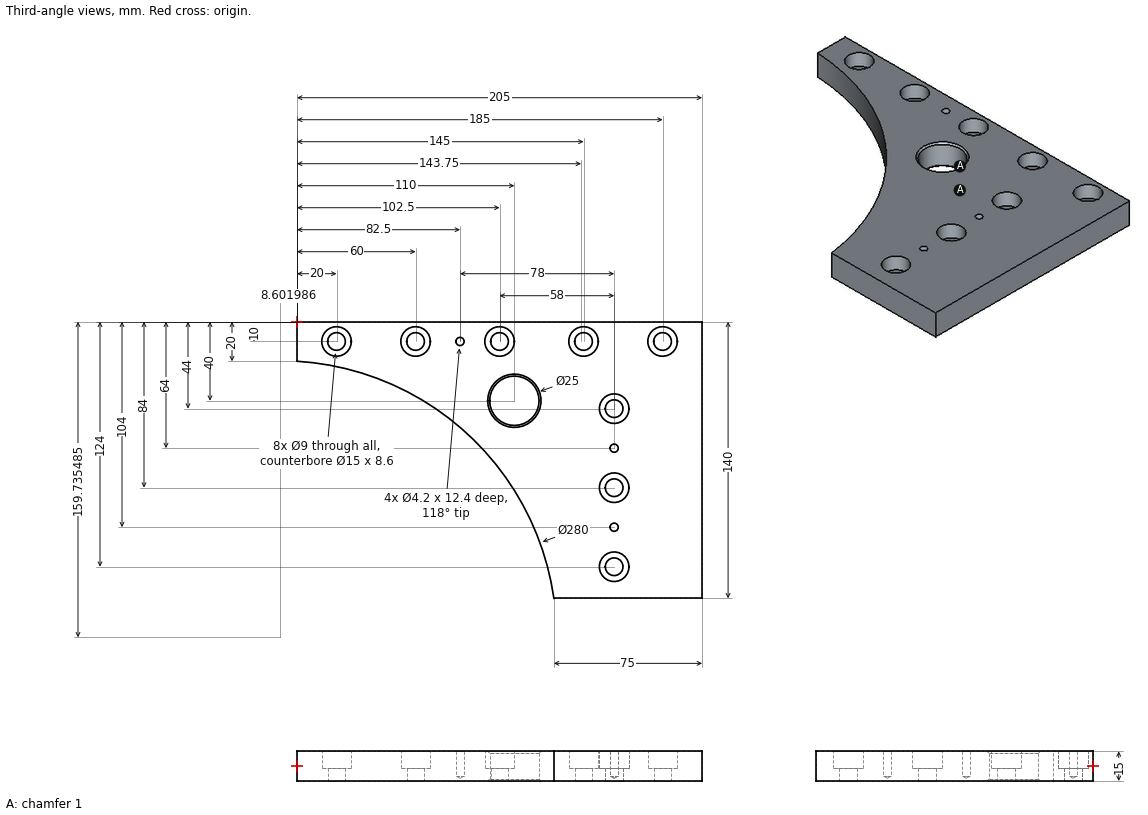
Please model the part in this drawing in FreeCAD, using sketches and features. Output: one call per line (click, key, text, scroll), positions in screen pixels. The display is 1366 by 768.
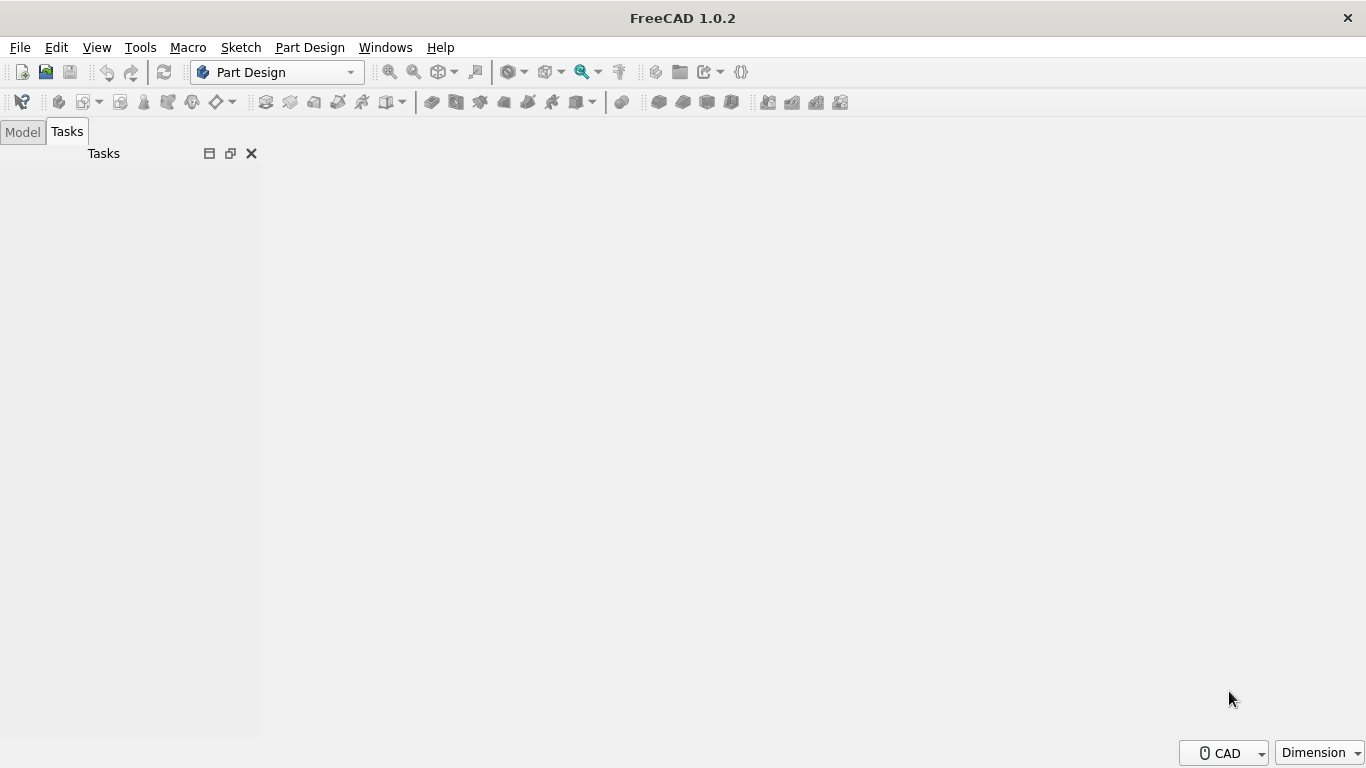
click(22, 72)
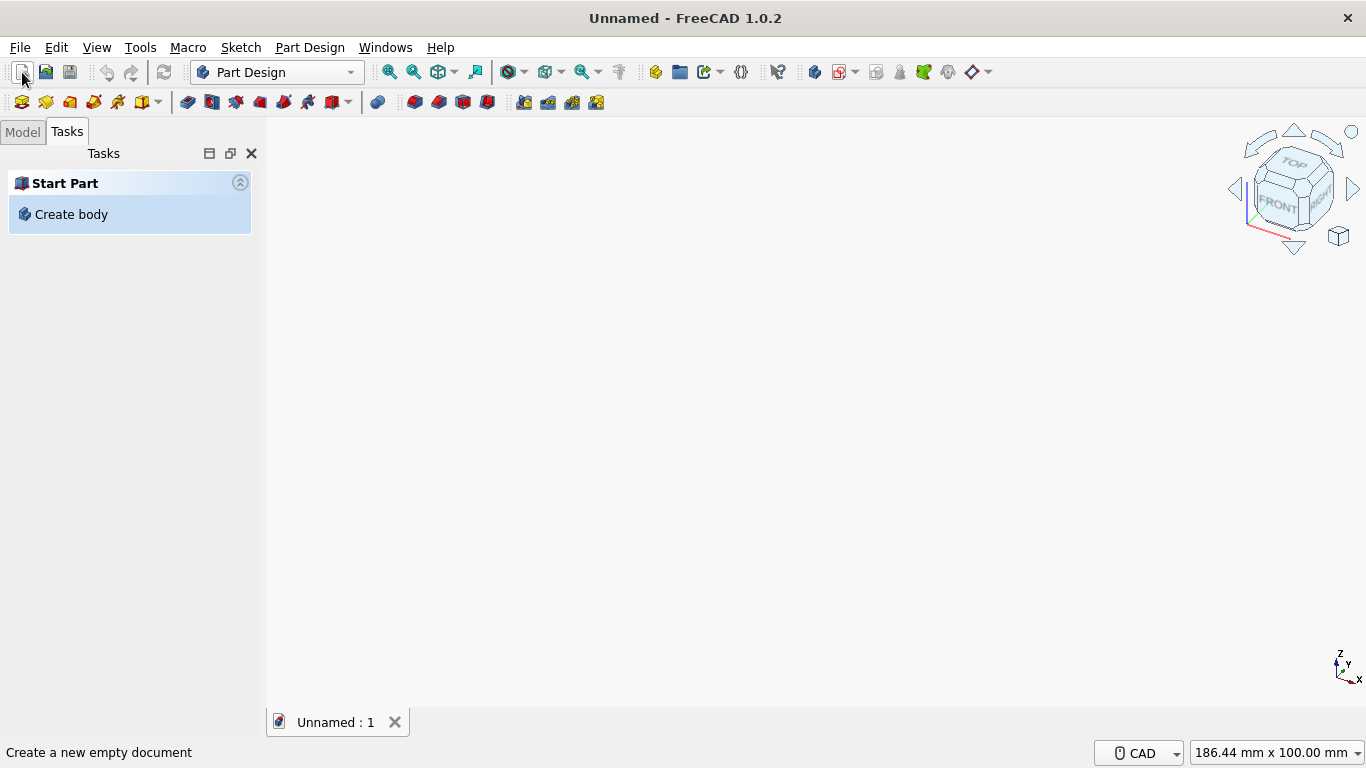
click(840, 72)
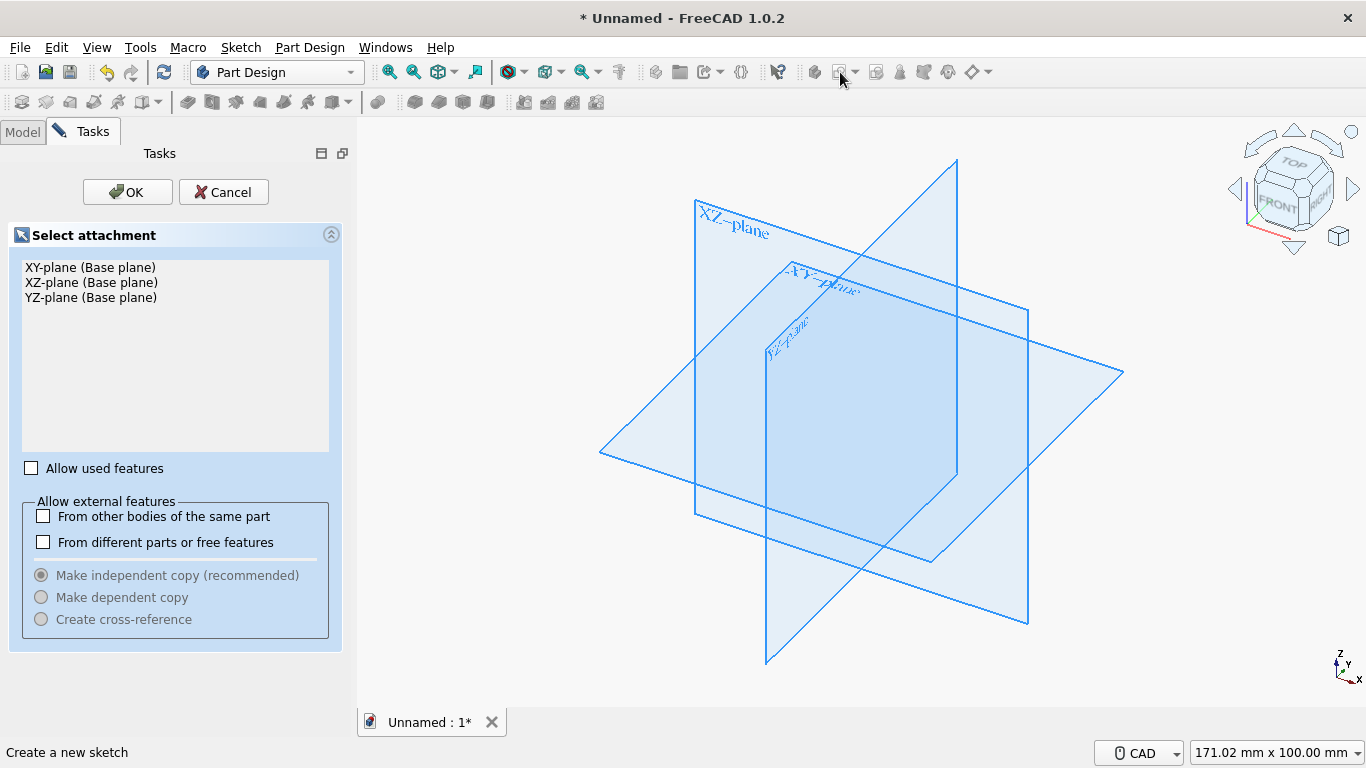
click(82, 268)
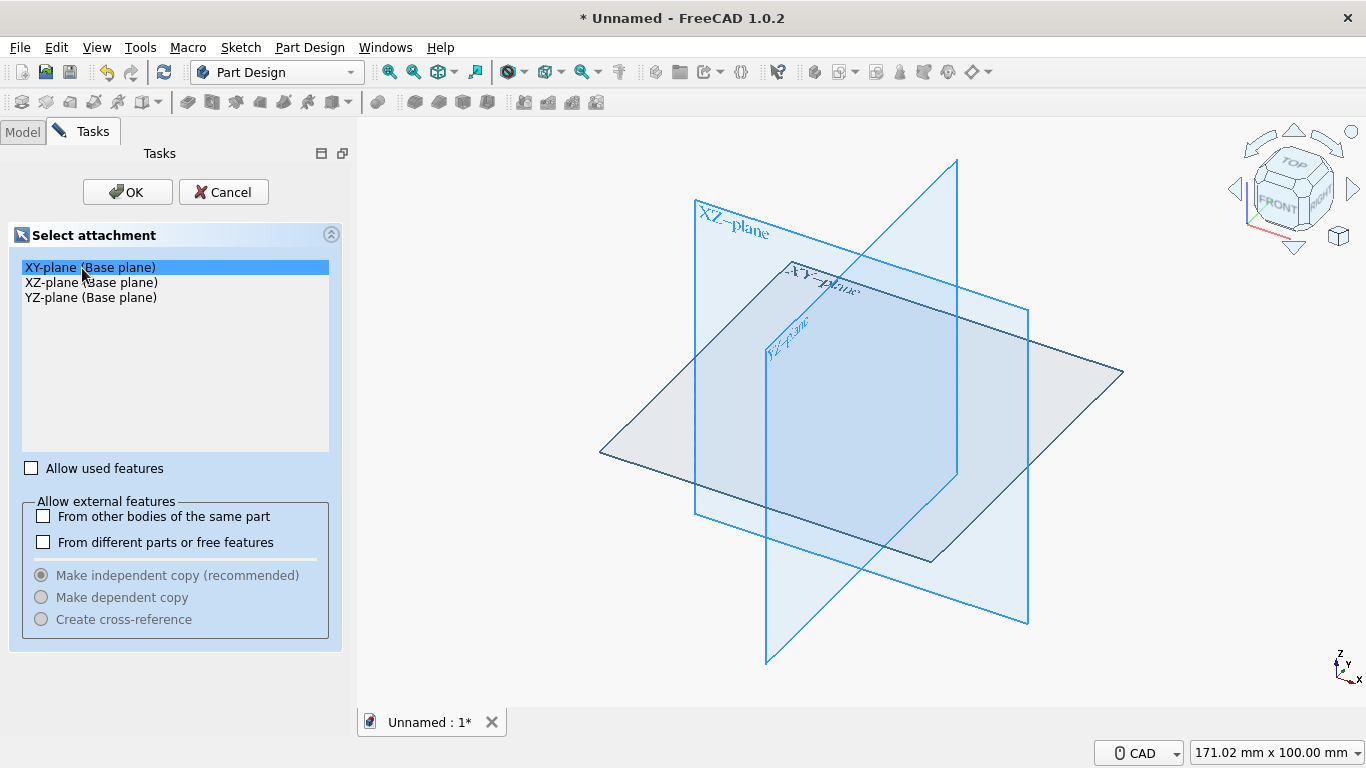
click(128, 192)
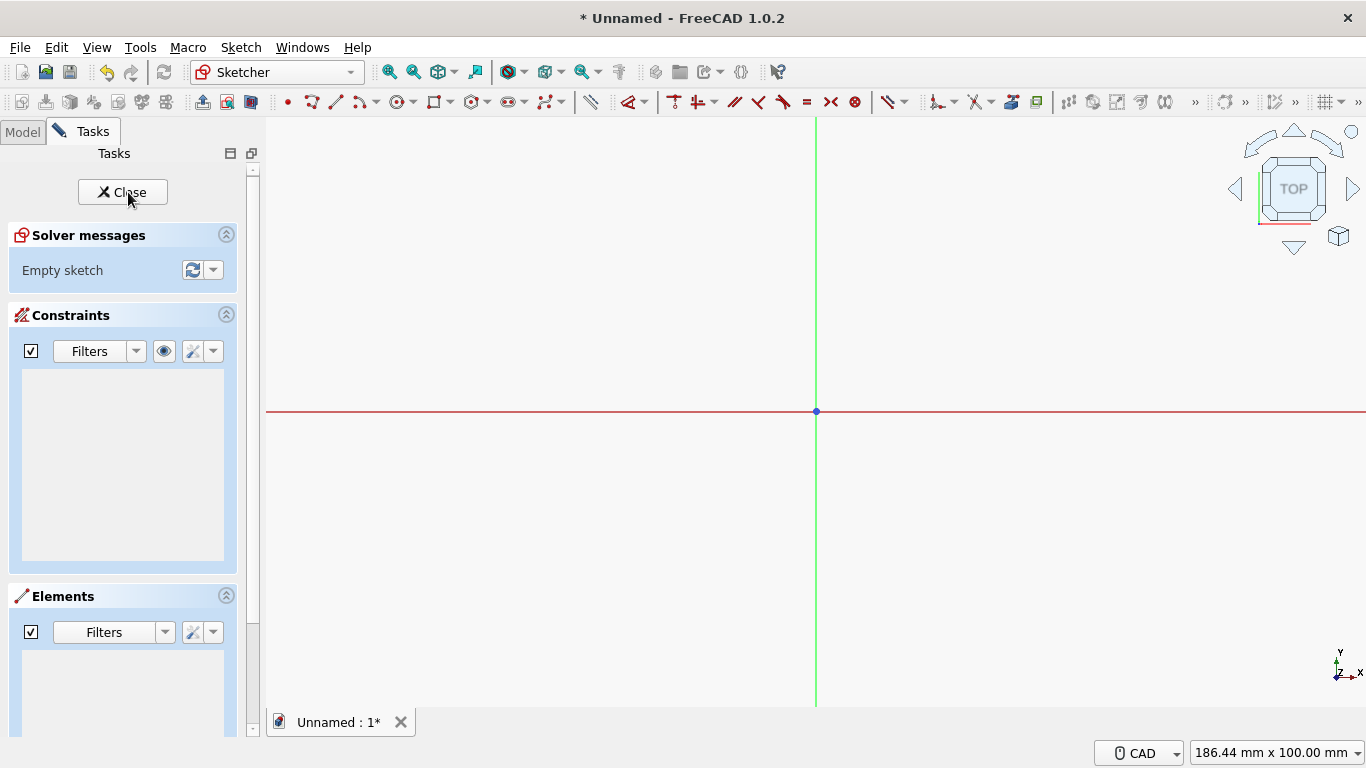
scroll(294, 145, down, 4)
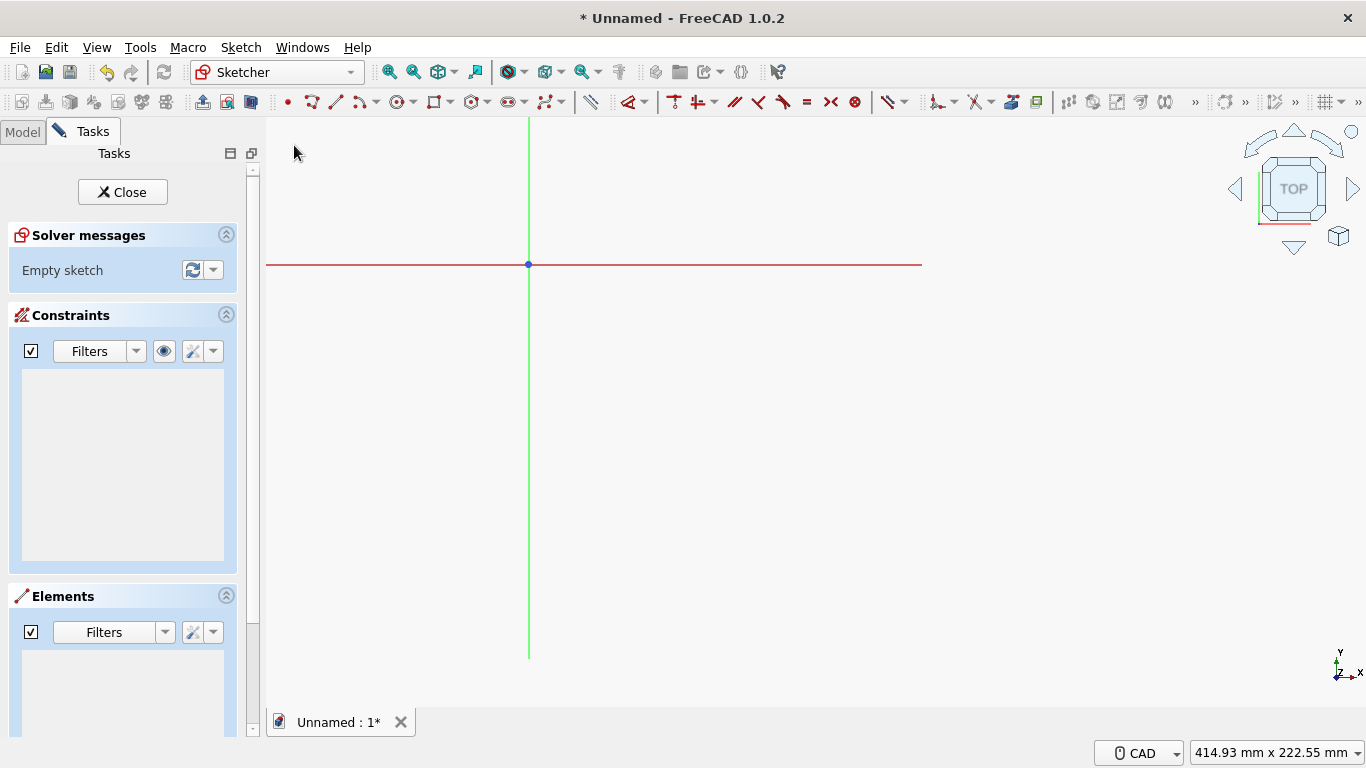
click(312, 102)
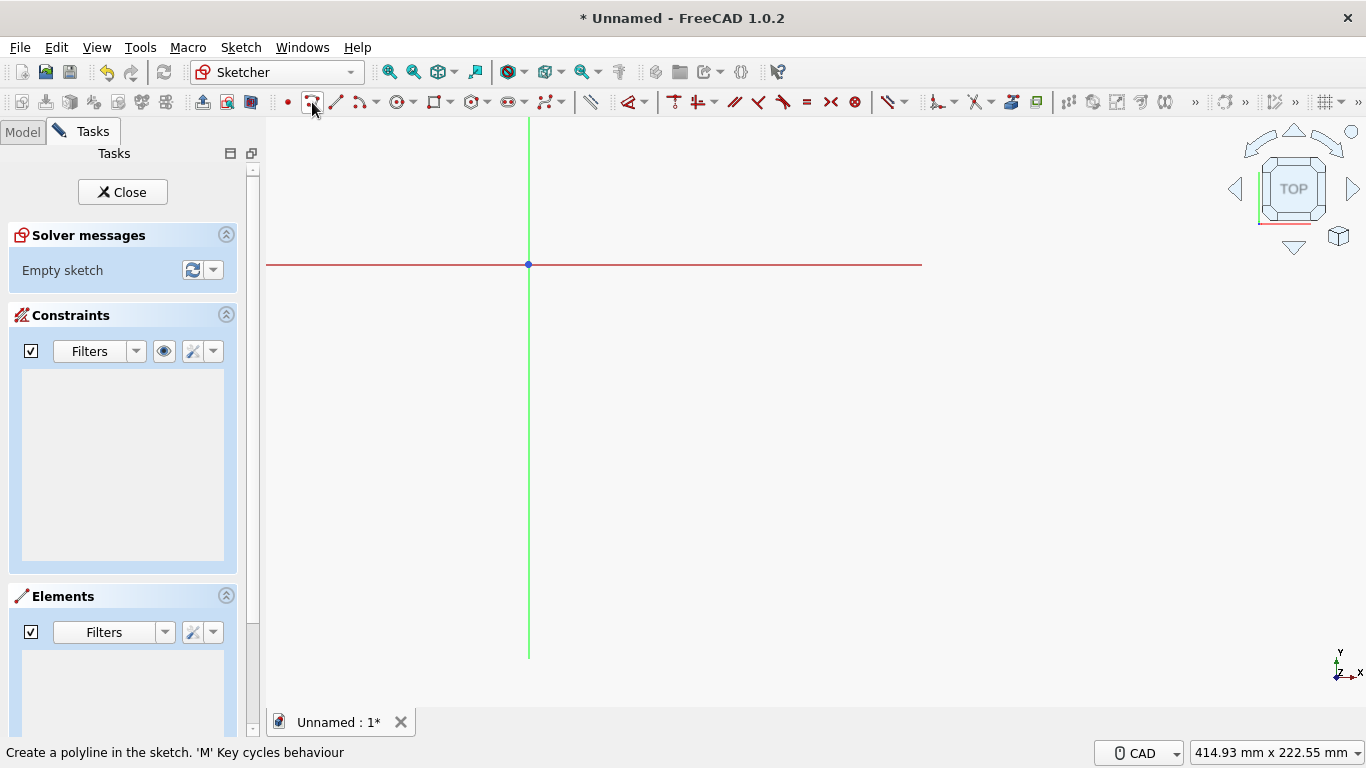
click(529, 265)
click(538, 318)
click(873, 636)
click(1072, 636)
click(1072, 274)
click(529, 265)
key(Escape)
key(Escape)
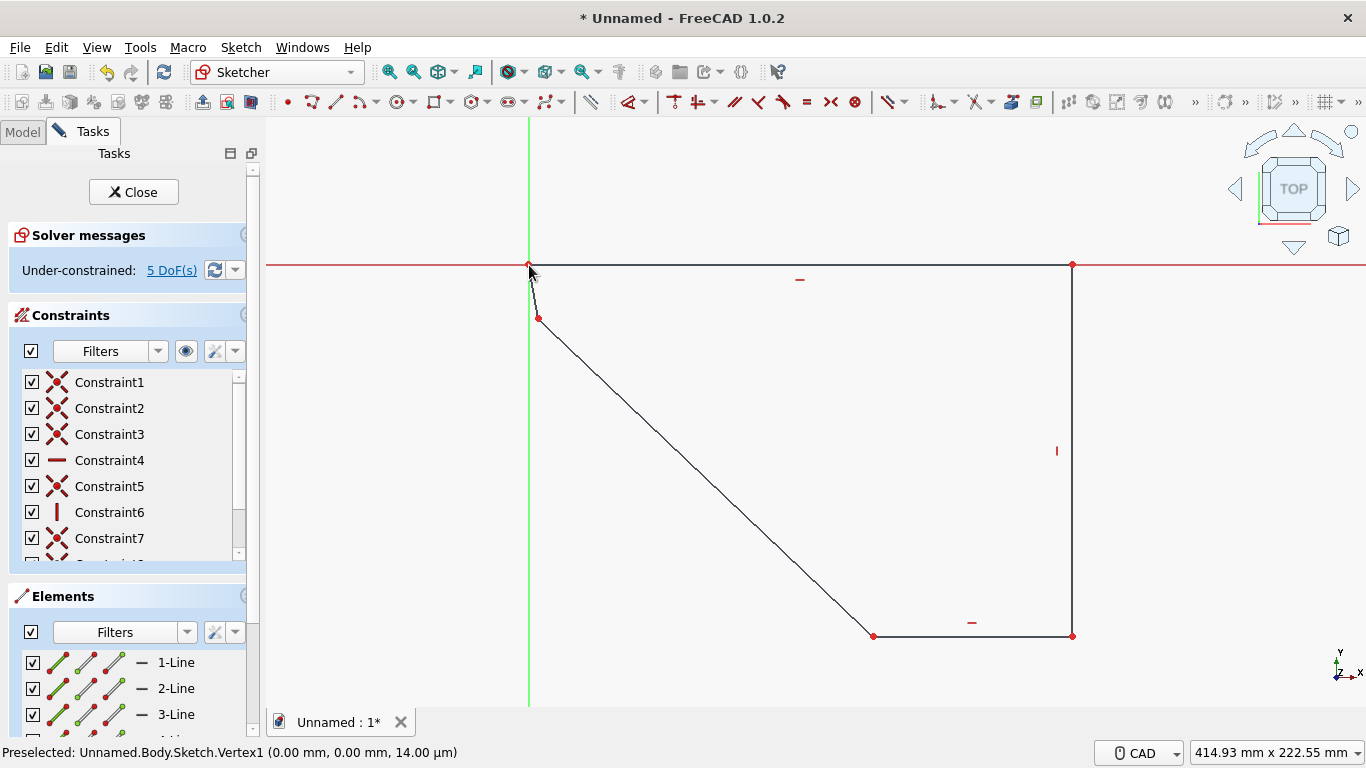
click(531, 281)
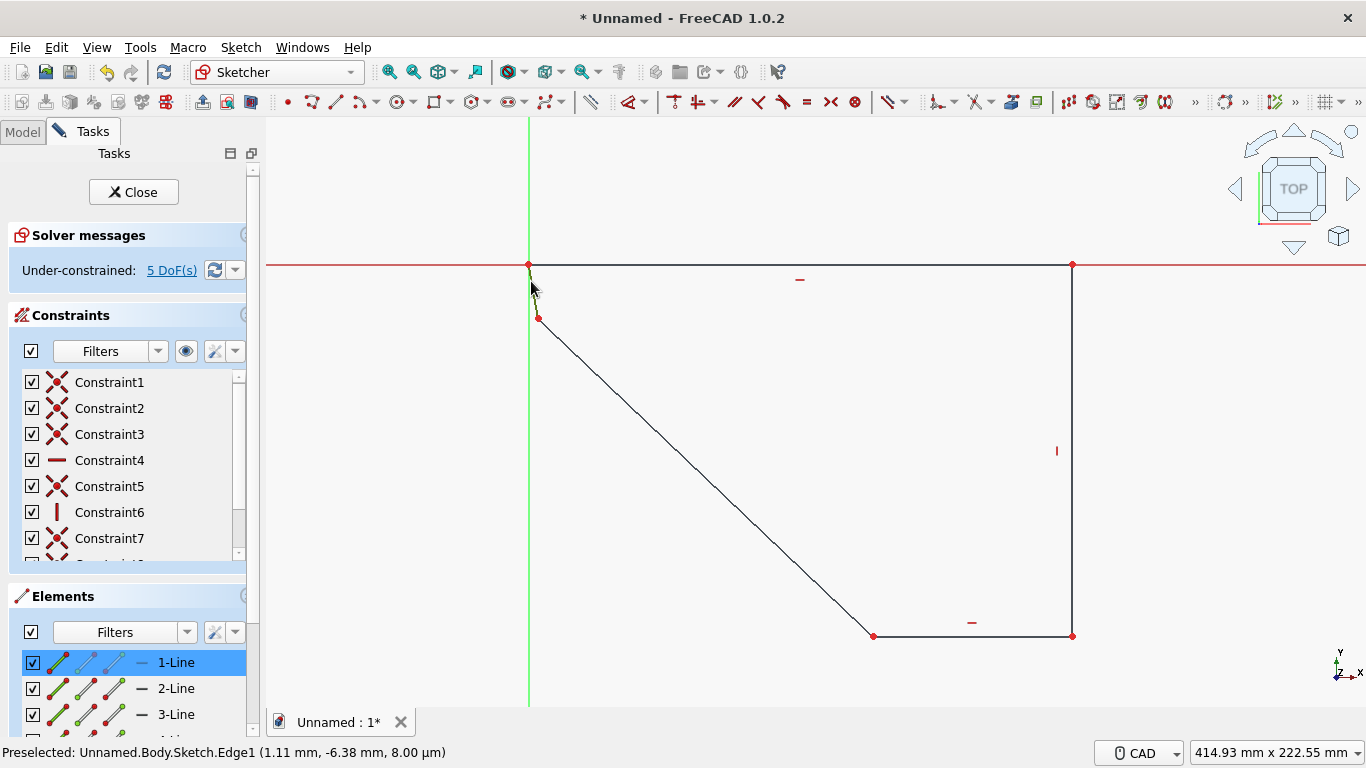
click(716, 102)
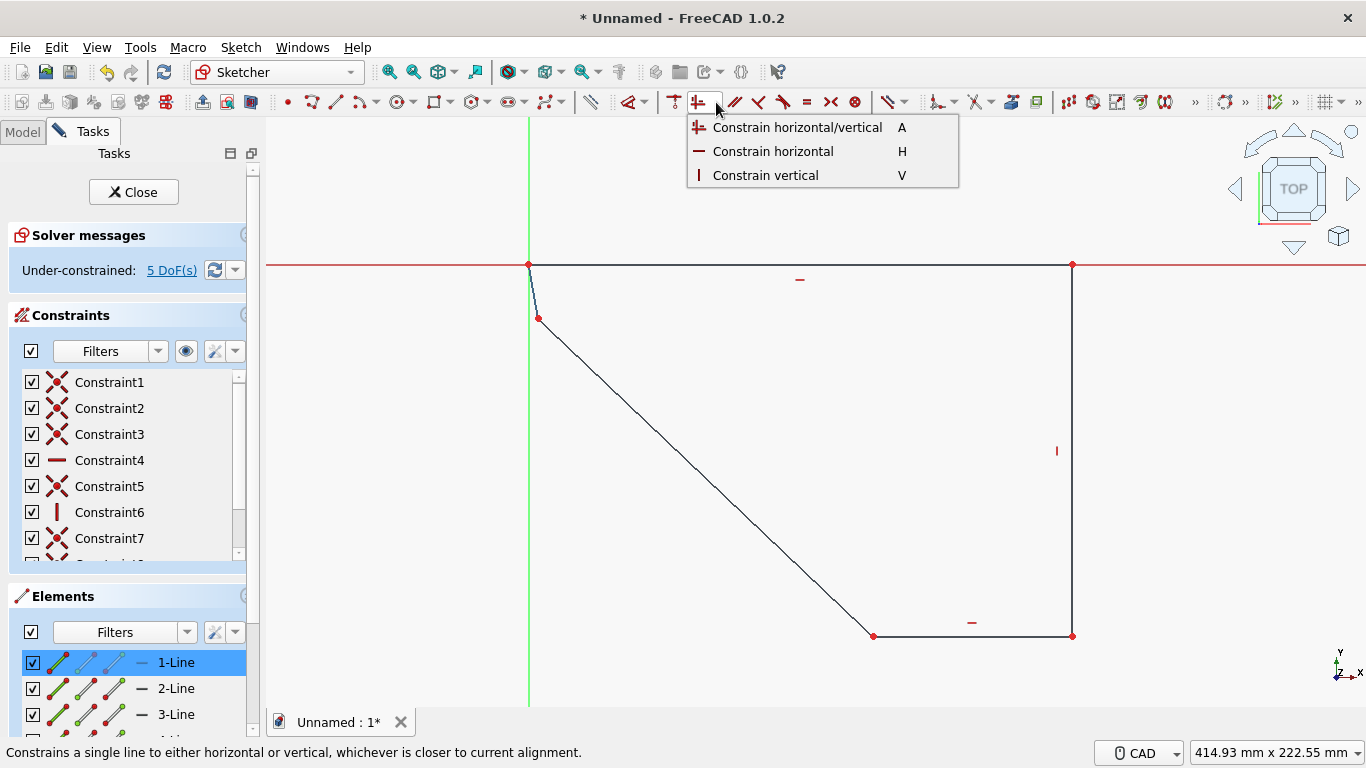
click(823, 175)